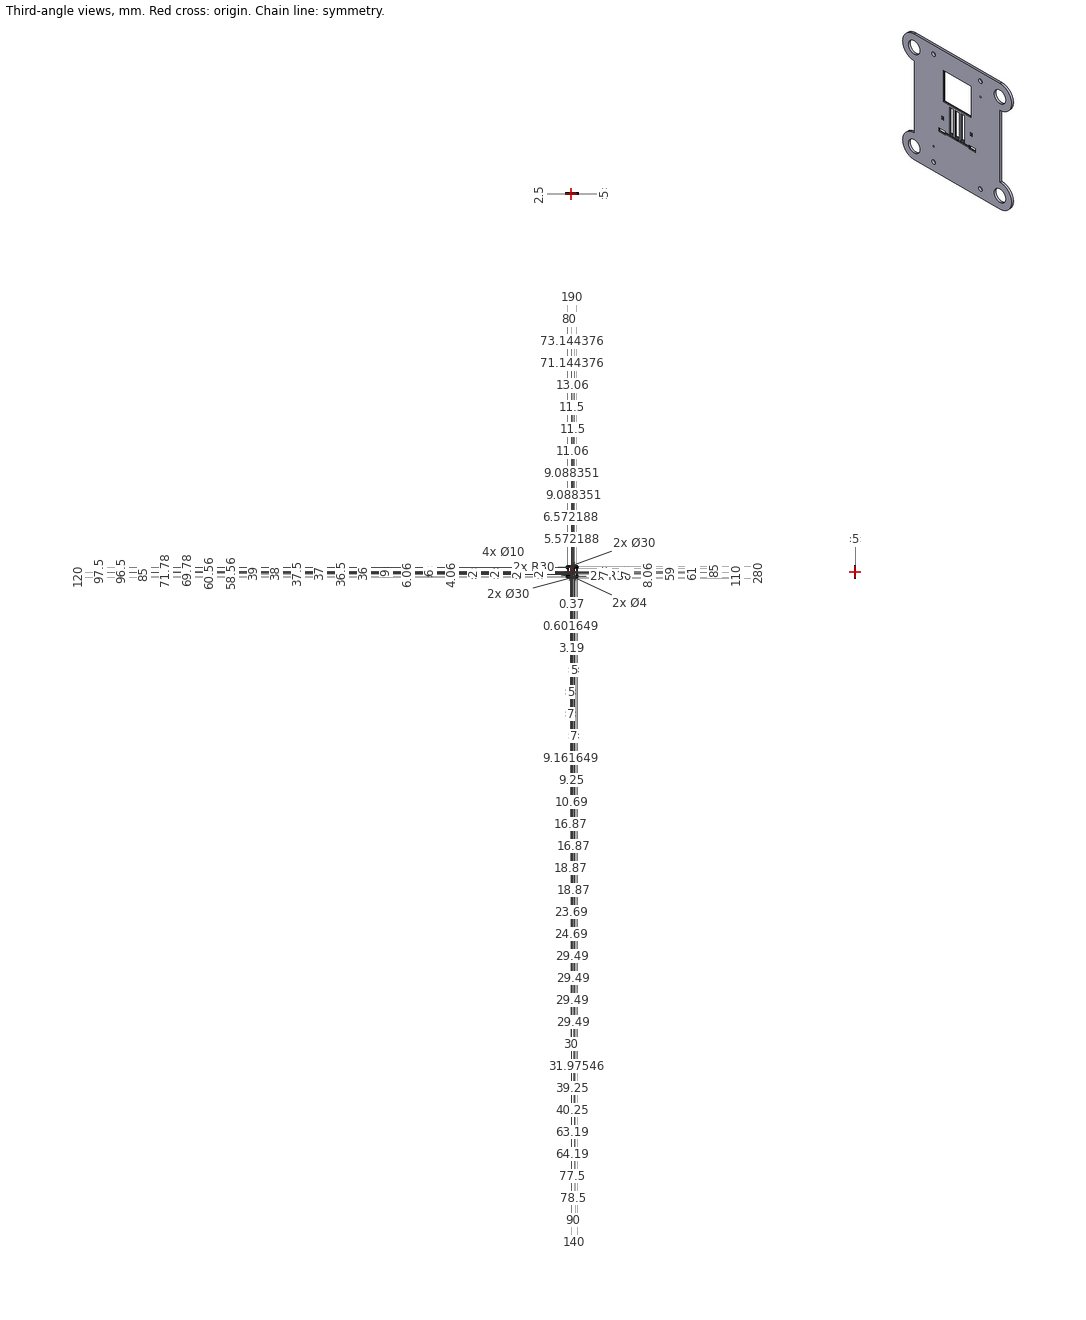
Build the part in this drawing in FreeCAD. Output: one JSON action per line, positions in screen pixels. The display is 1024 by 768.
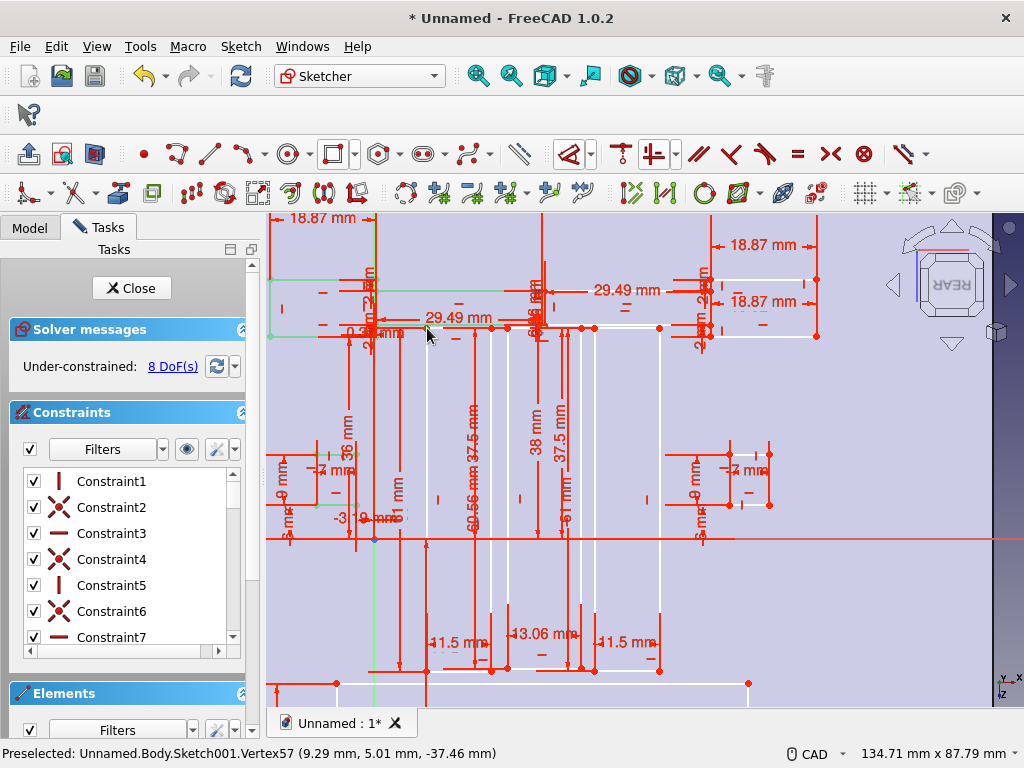
{"action": "left_click", "coordinate": [590, 154]}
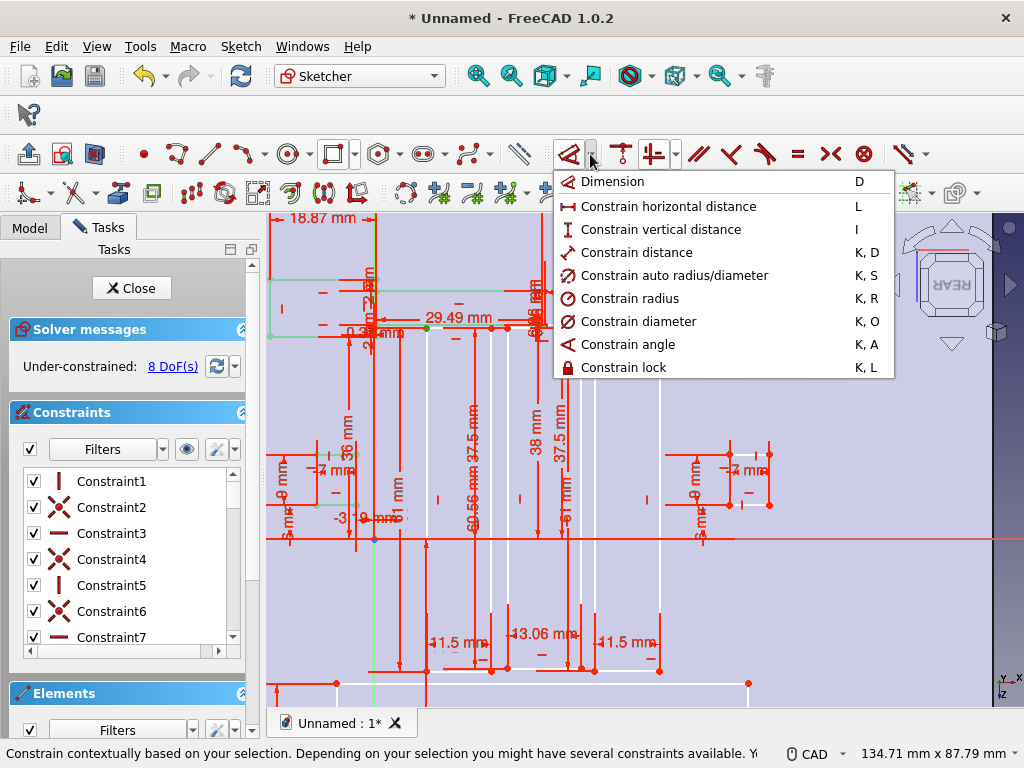
{"action": "left_click", "coordinate": [724, 206]}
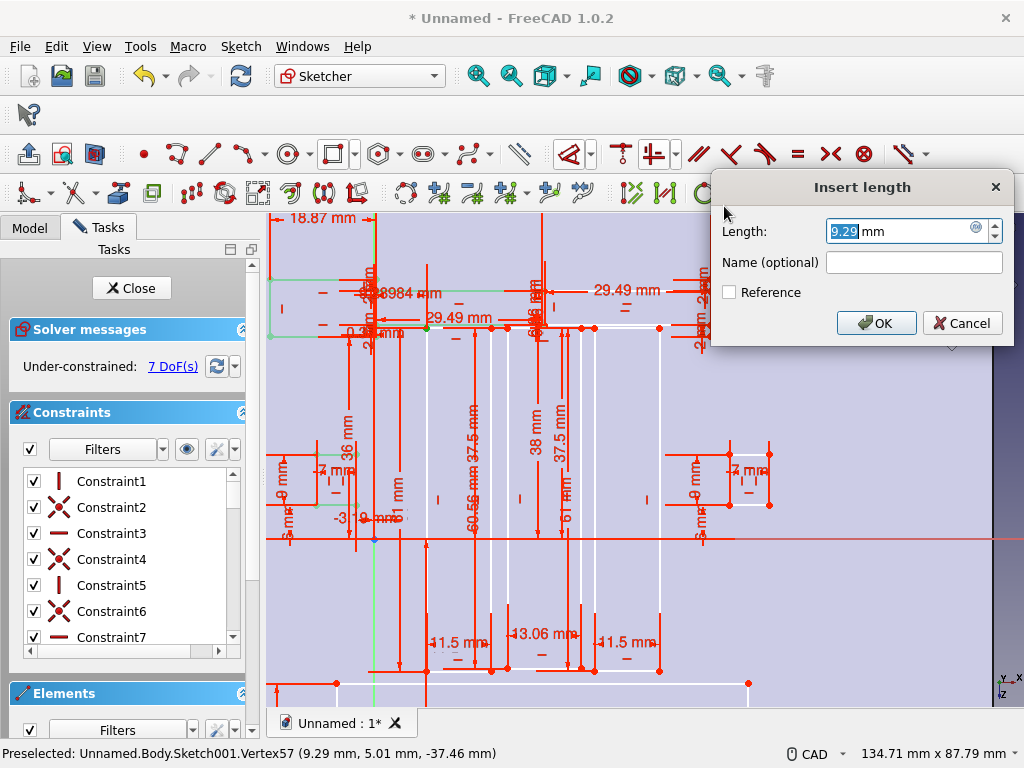
{"action": "type", "text": "9.25"}
{"action": "key", "text": "Return"}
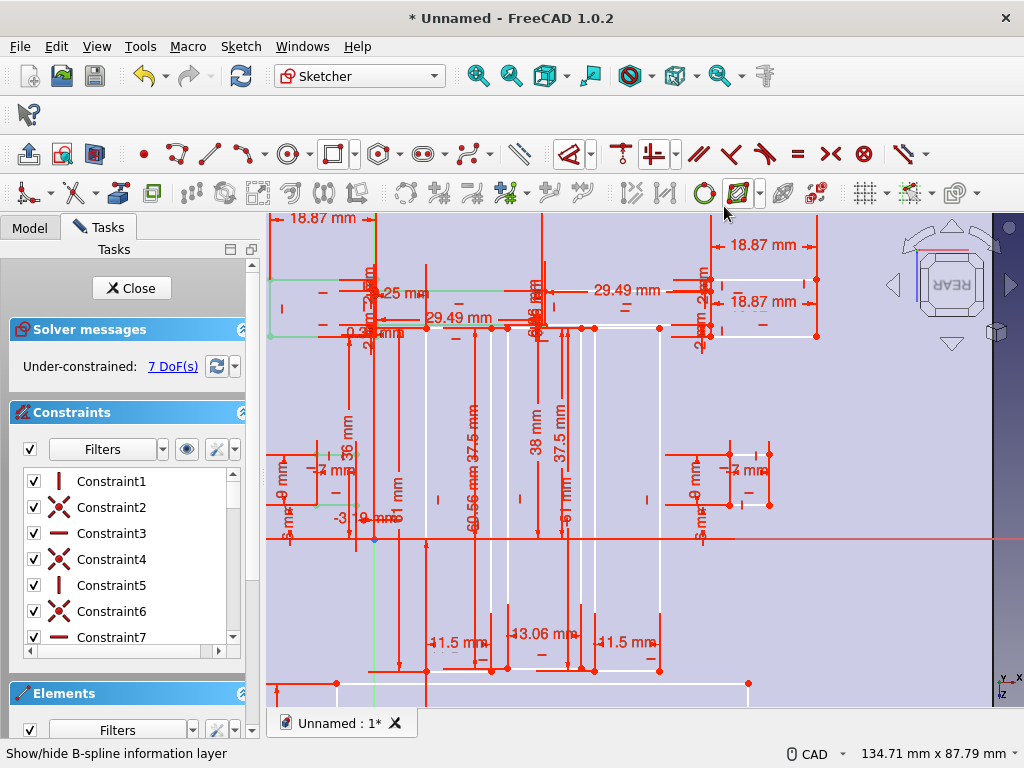
{"action": "left_click", "coordinate": [426, 328]}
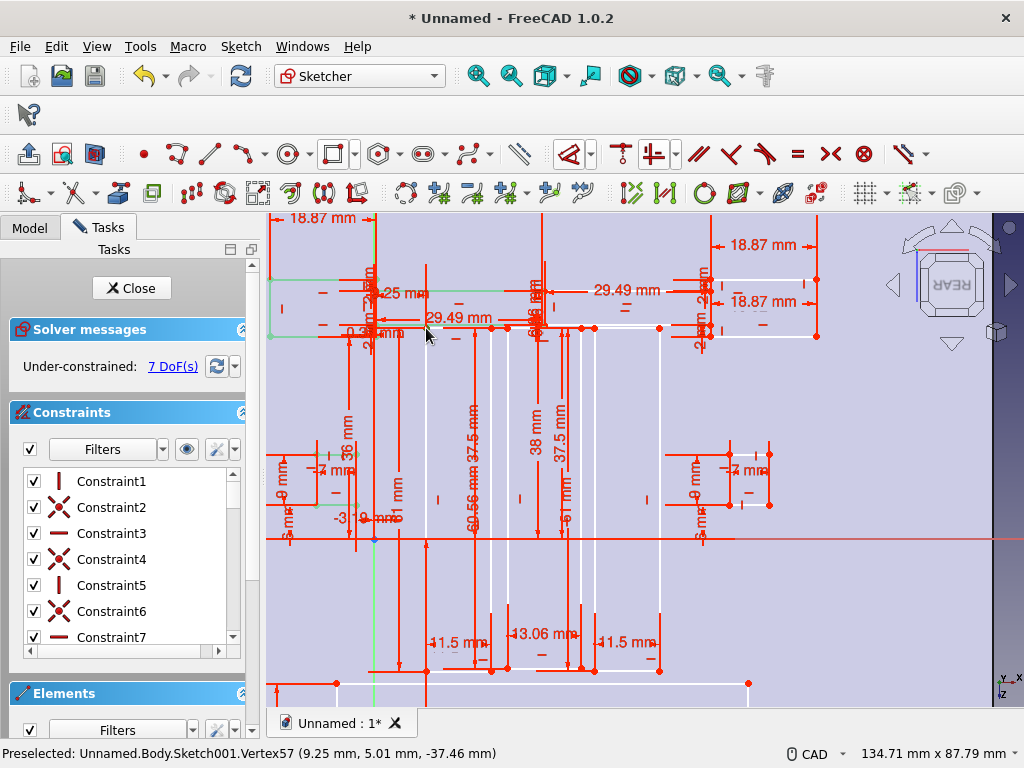
{"action": "left_click", "coordinate": [590, 154]}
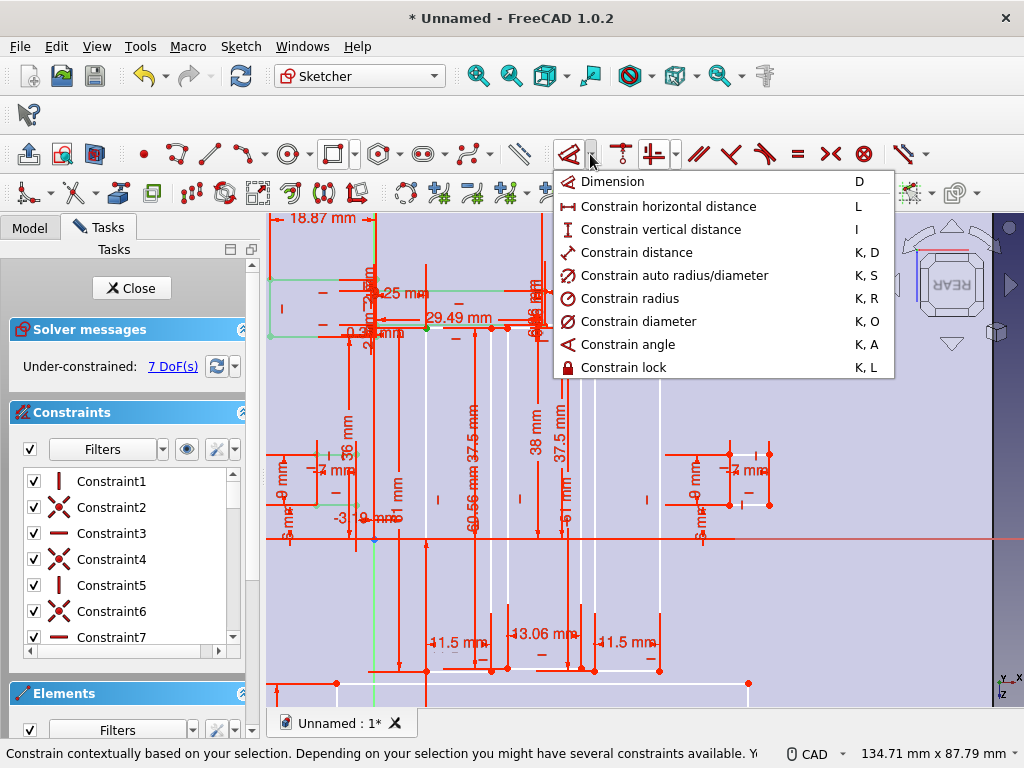
{"action": "left_click", "coordinate": [724, 230]}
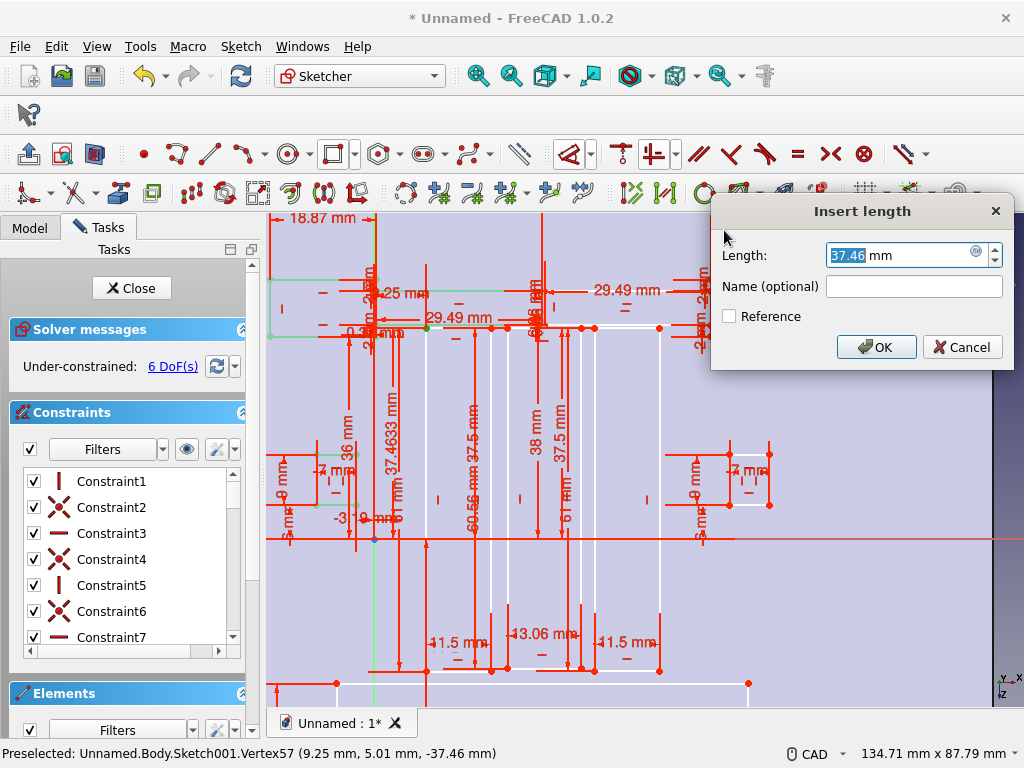
{"action": "type", "text": "37.5"}
{"action": "key", "text": "Return"}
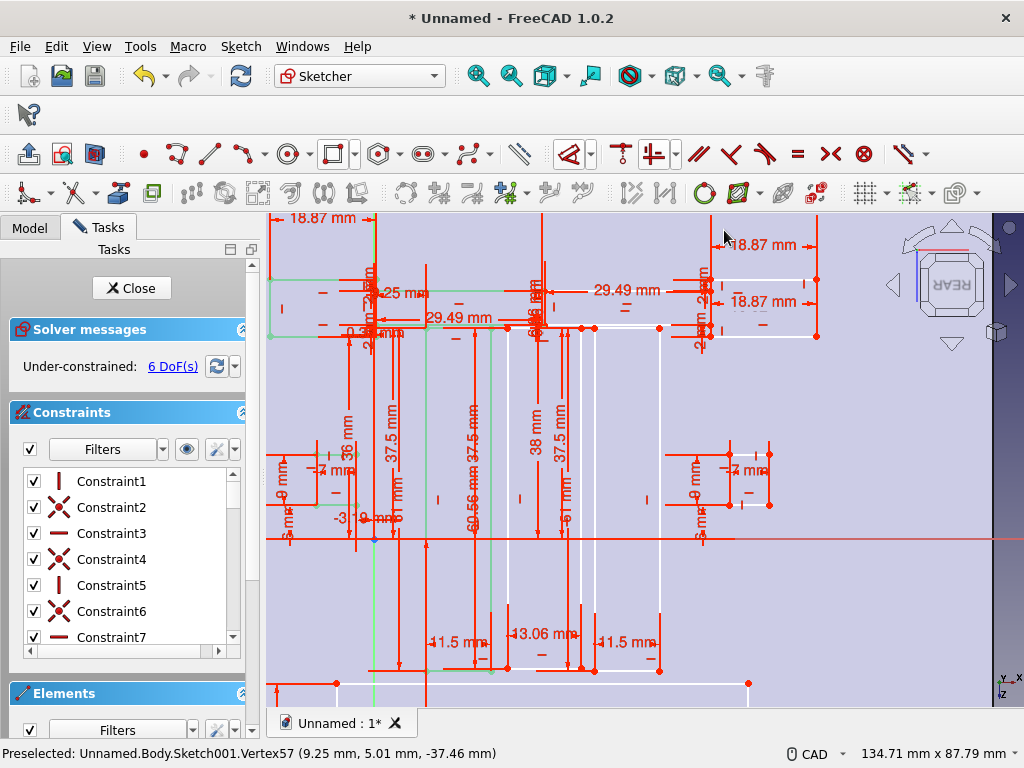
{"action": "left_click", "coordinate": [817, 337]}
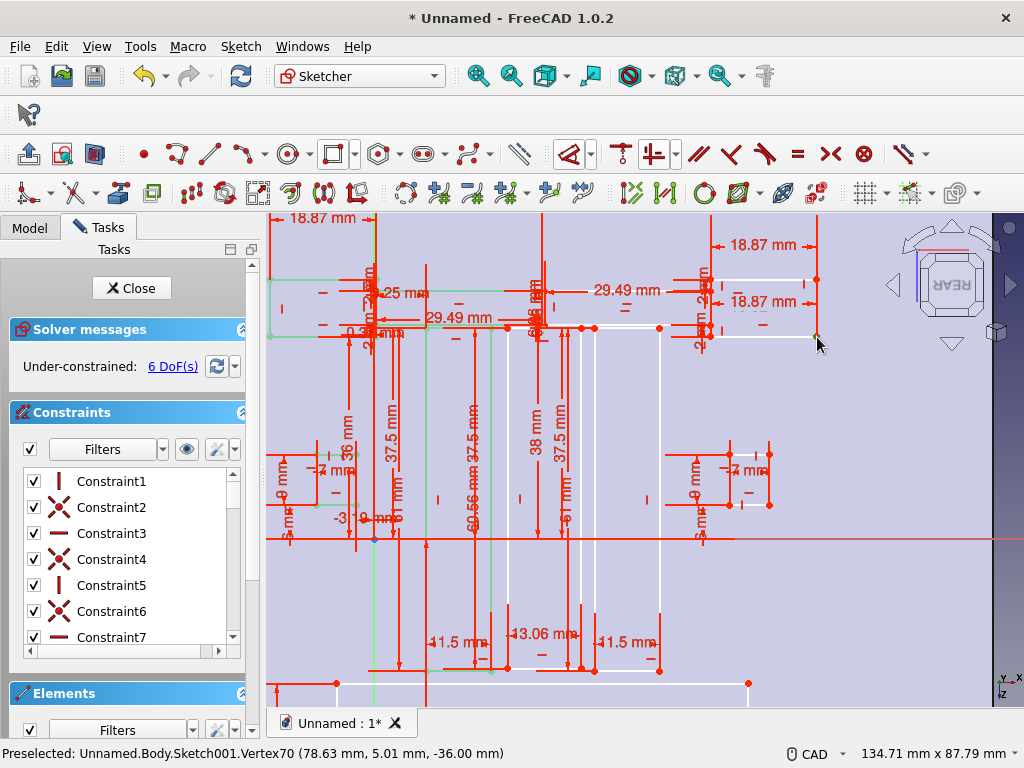
{"action": "left_click", "coordinate": [590, 154]}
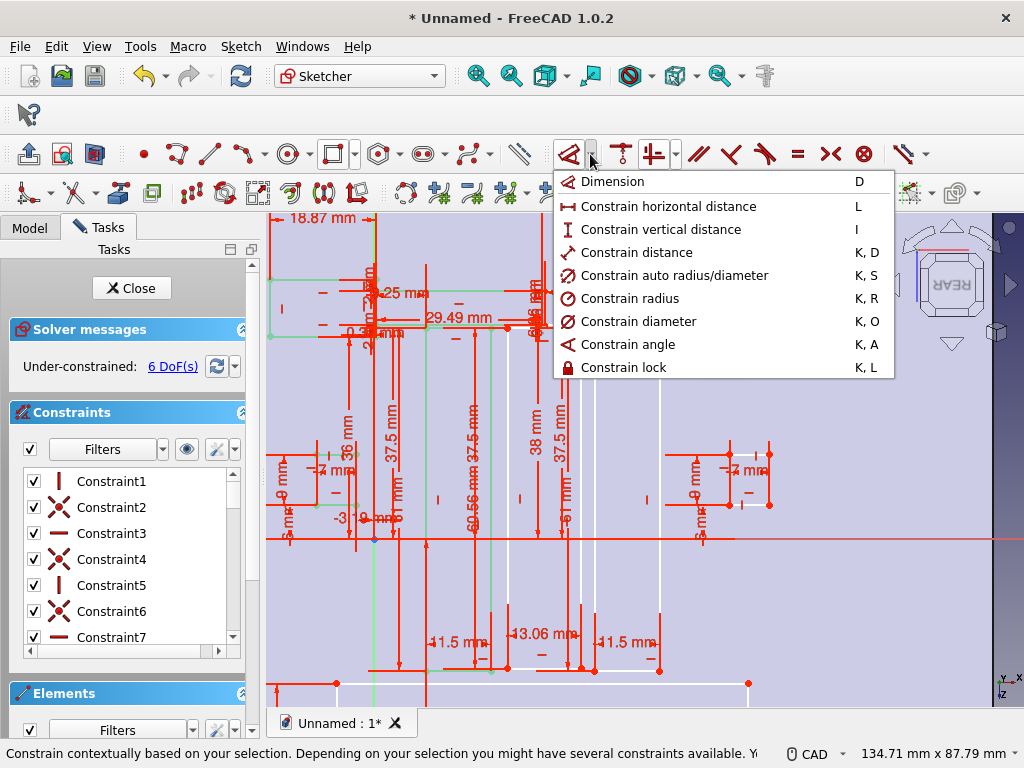
{"action": "left_click", "coordinate": [724, 206]}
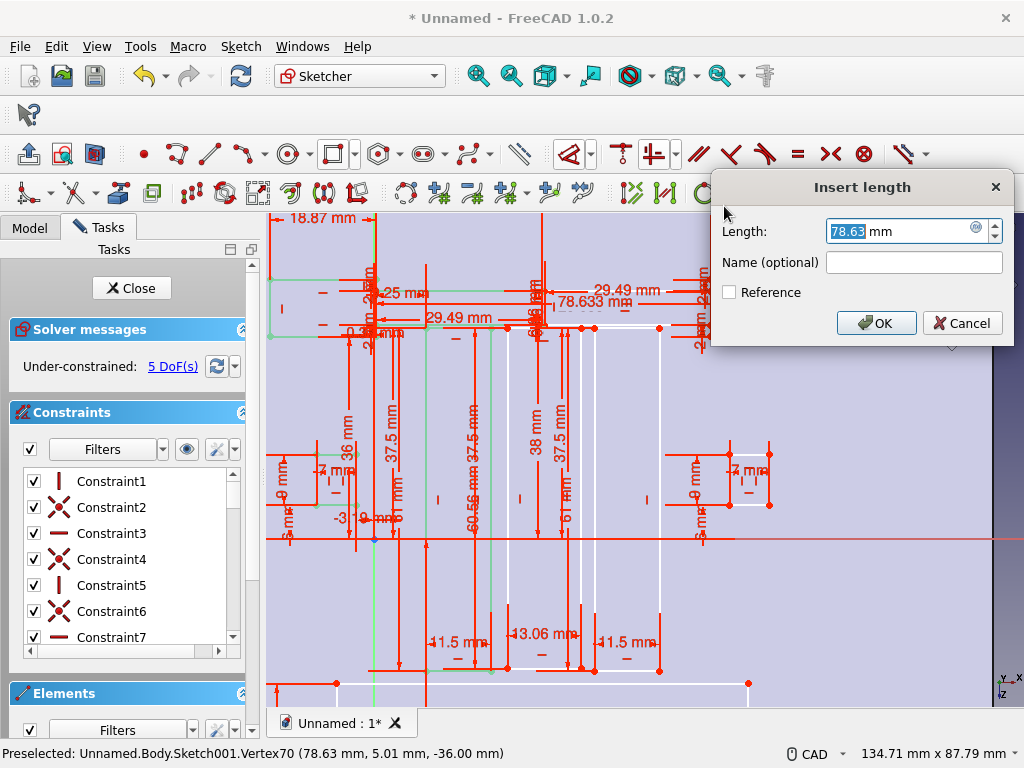
{"action": "type", "text": "78.5"}
{"action": "key", "text": "Return"}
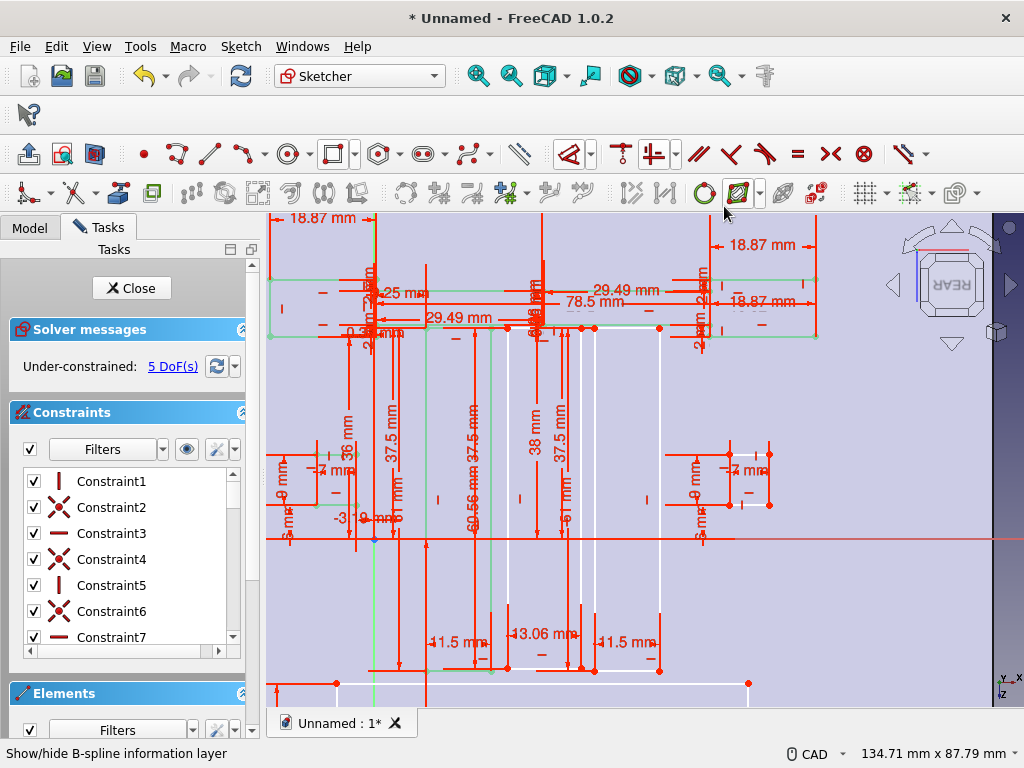
{"action": "left_click", "coordinate": [730, 455]}